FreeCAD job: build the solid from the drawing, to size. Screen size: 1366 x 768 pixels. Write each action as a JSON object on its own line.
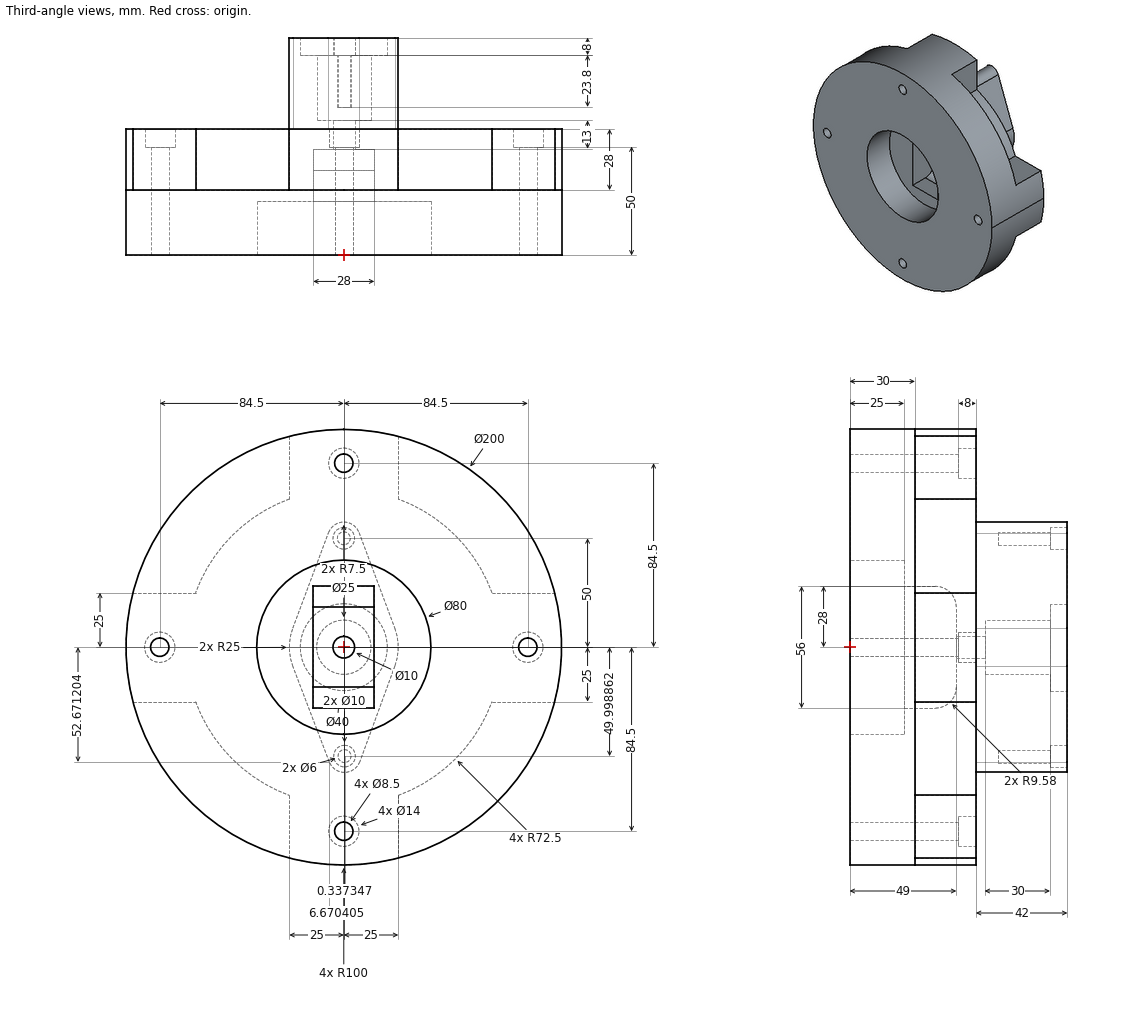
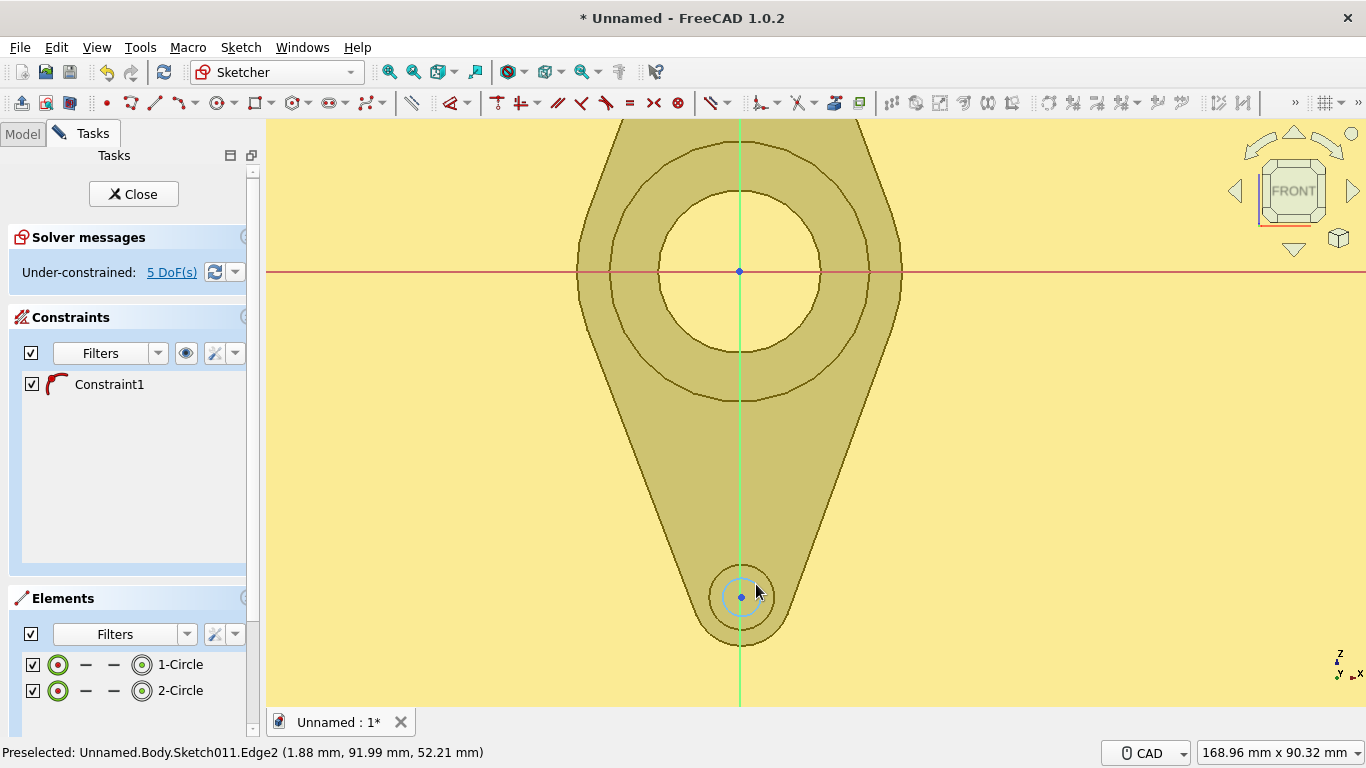
{"action": "left_click", "coordinate": [755, 584]}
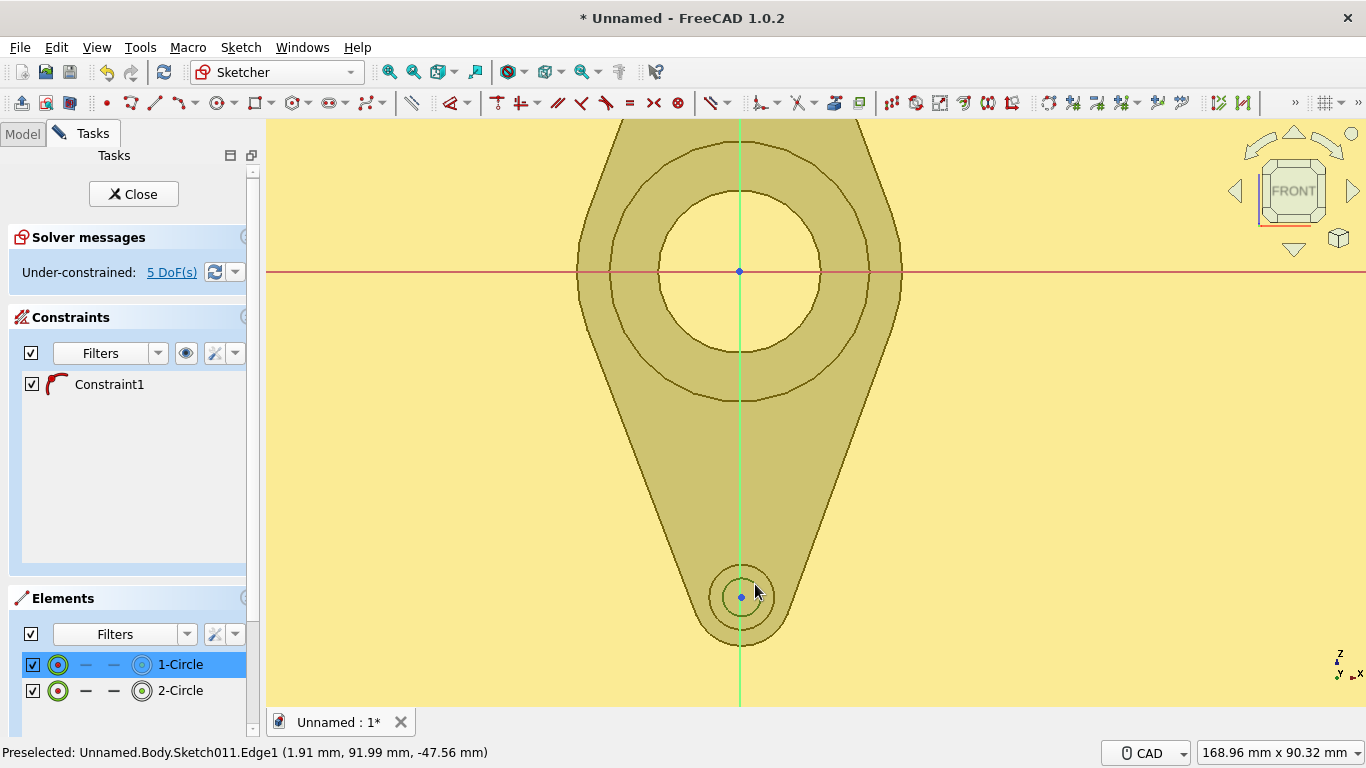
{"action": "scroll", "coordinate": [756, 585], "scroll_direction": "down", "scroll_amount": 3}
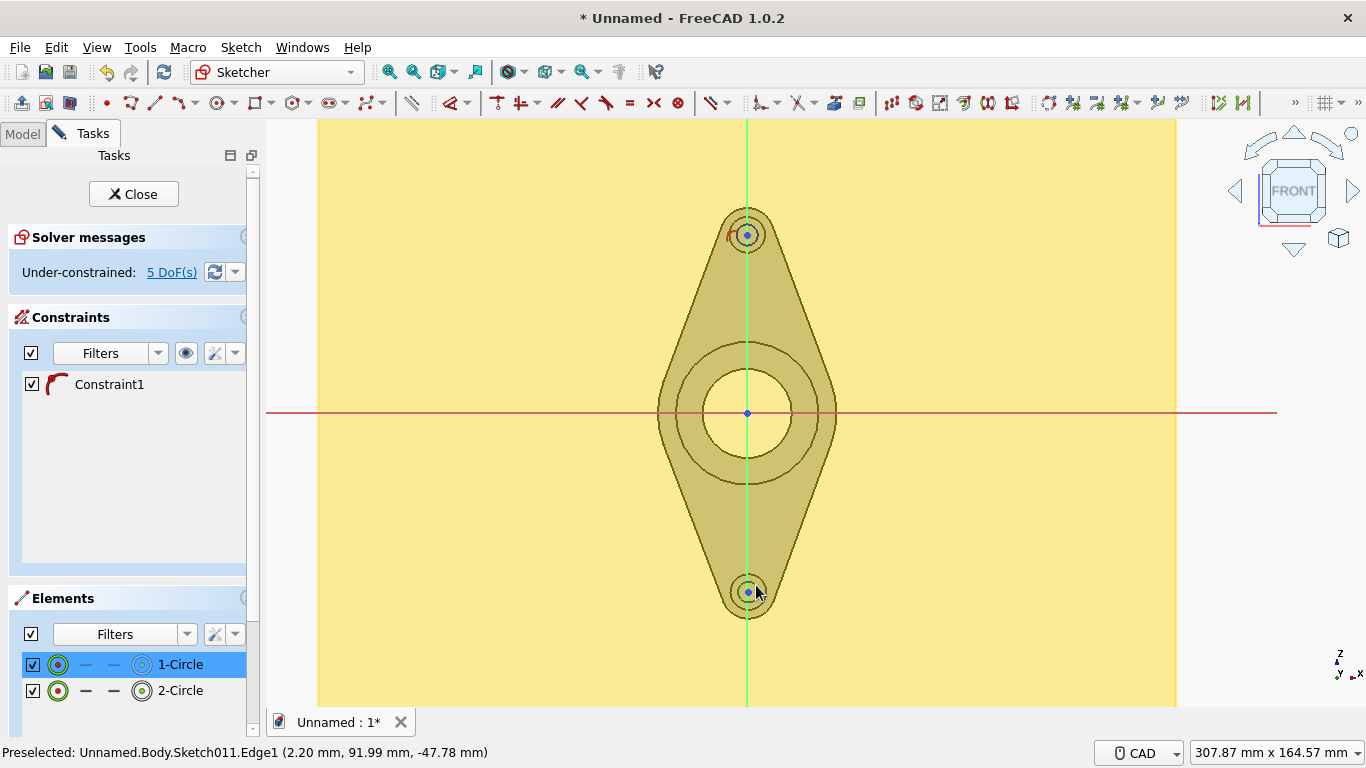
{"action": "scroll", "coordinate": [755, 228], "scroll_direction": "up", "scroll_amount": 4}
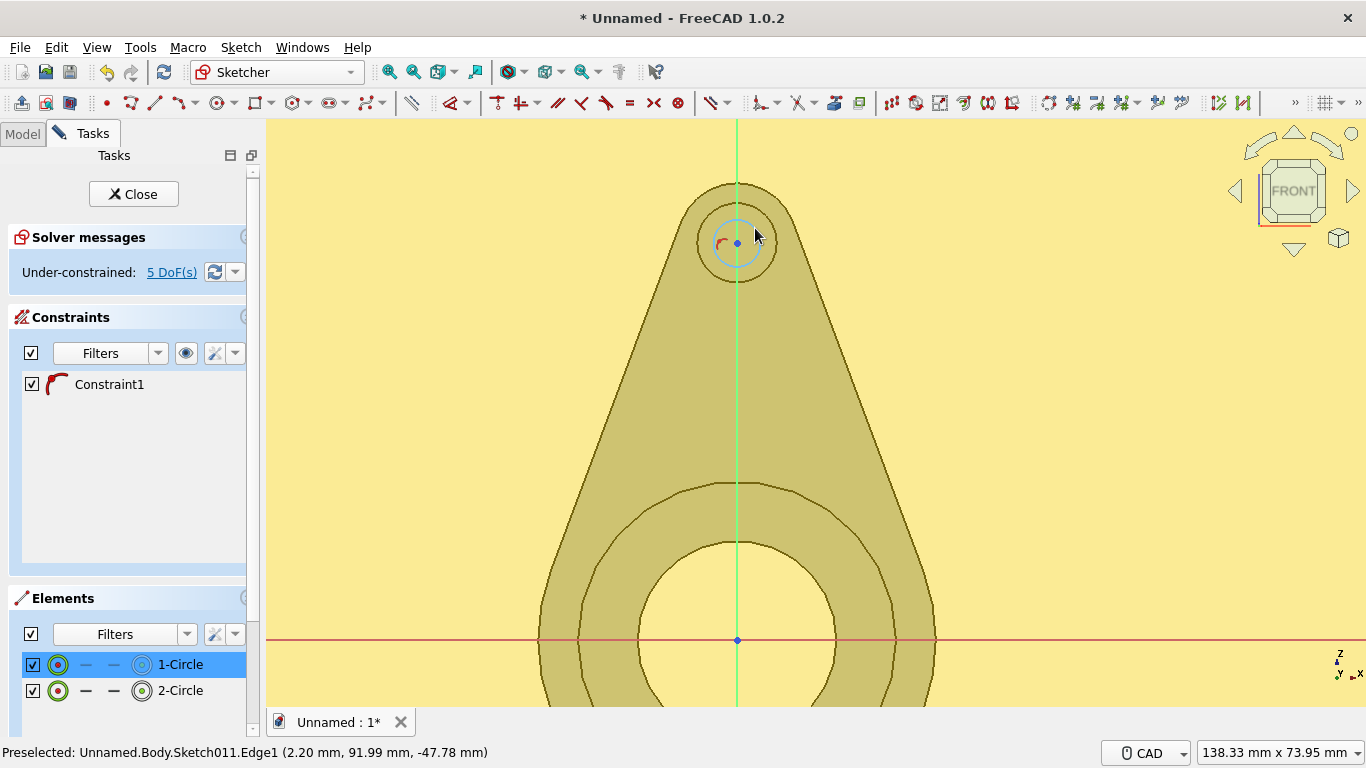
{"action": "left_click", "coordinate": [754, 227]}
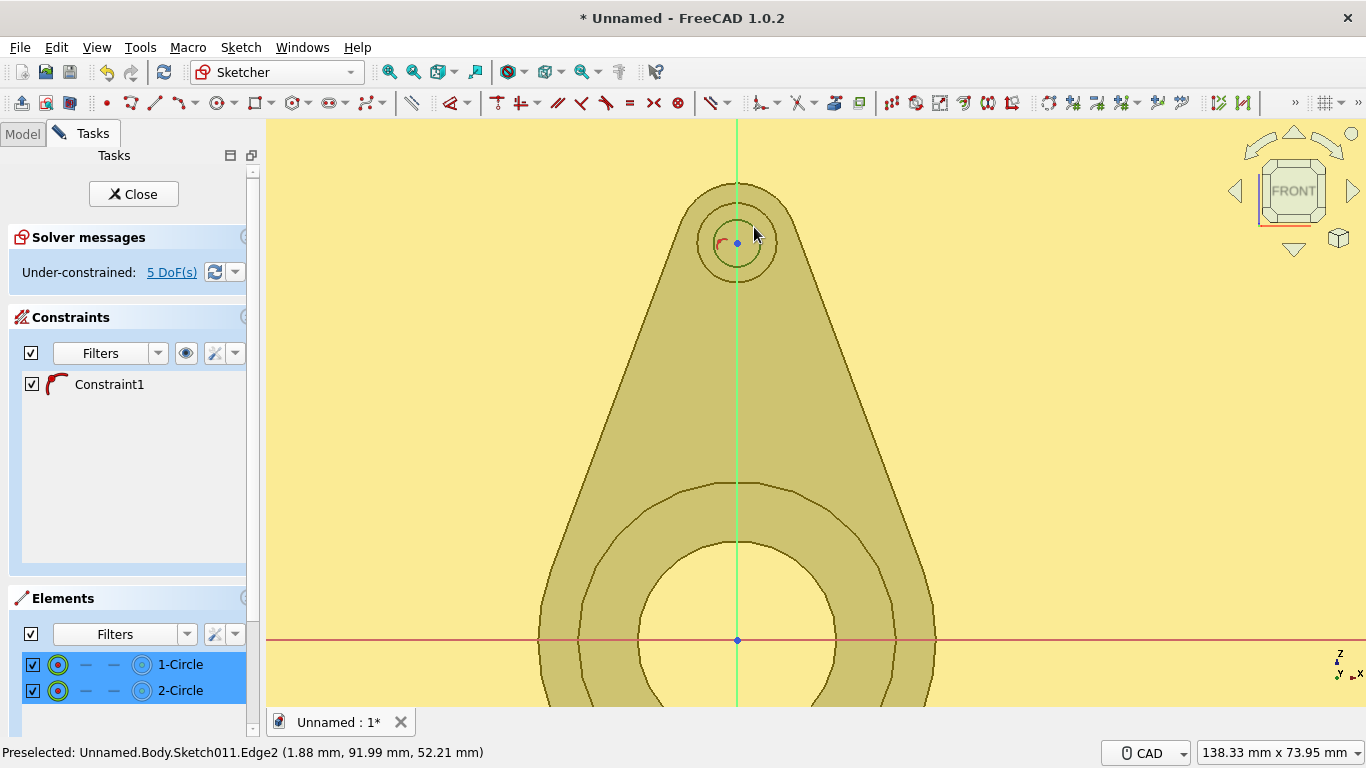
{"action": "left_click", "coordinate": [630, 104]}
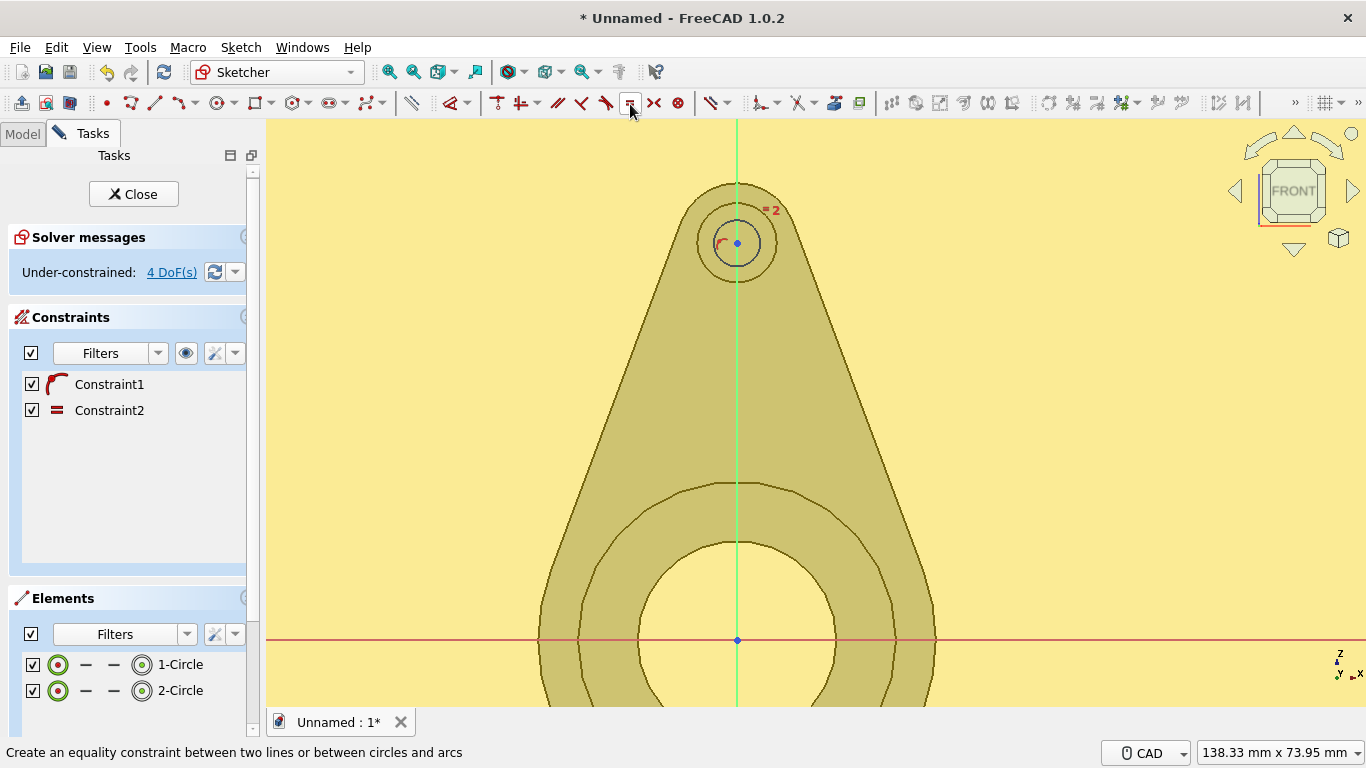
{"action": "key", "text": "d"}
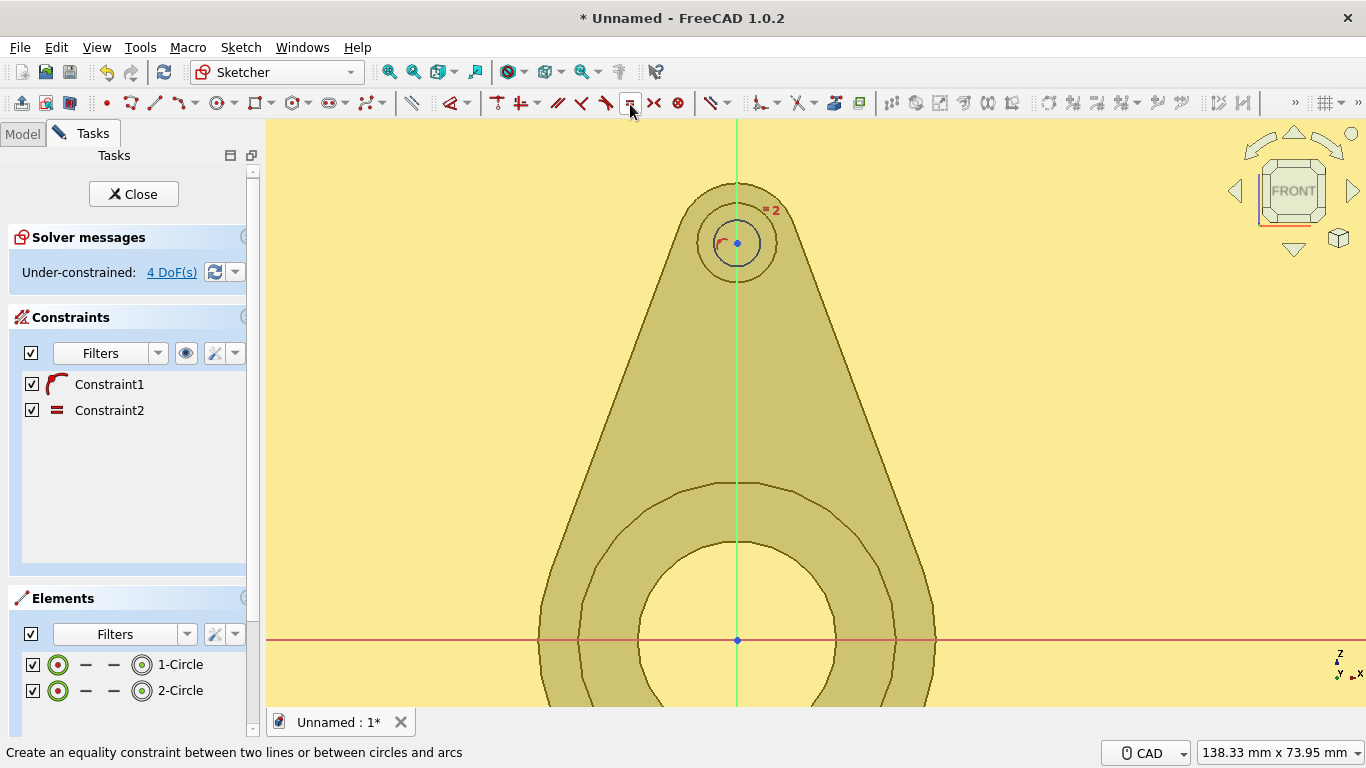
{"action": "scroll", "coordinate": [755, 227], "scroll_direction": "down", "scroll_amount": 4}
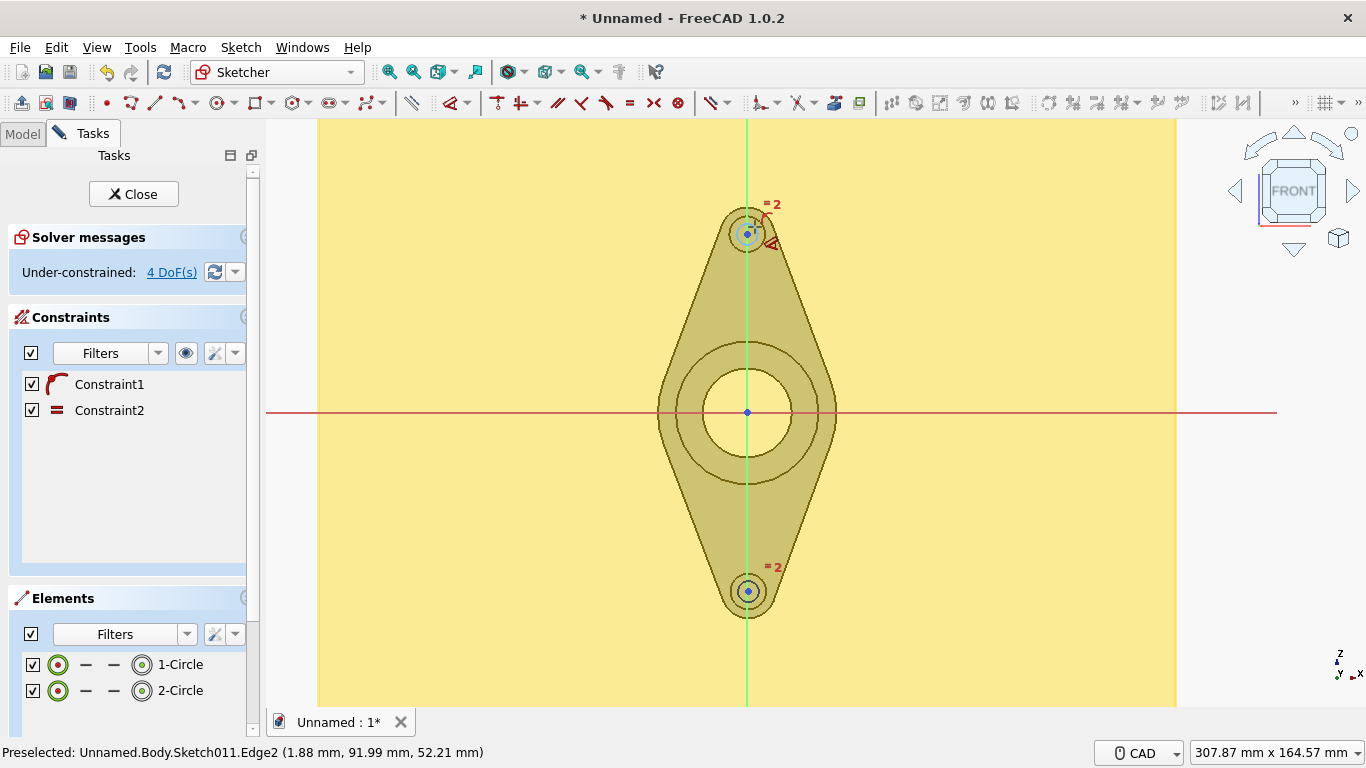
{"action": "scroll", "coordinate": [756, 584], "scroll_direction": "up", "scroll_amount": 4}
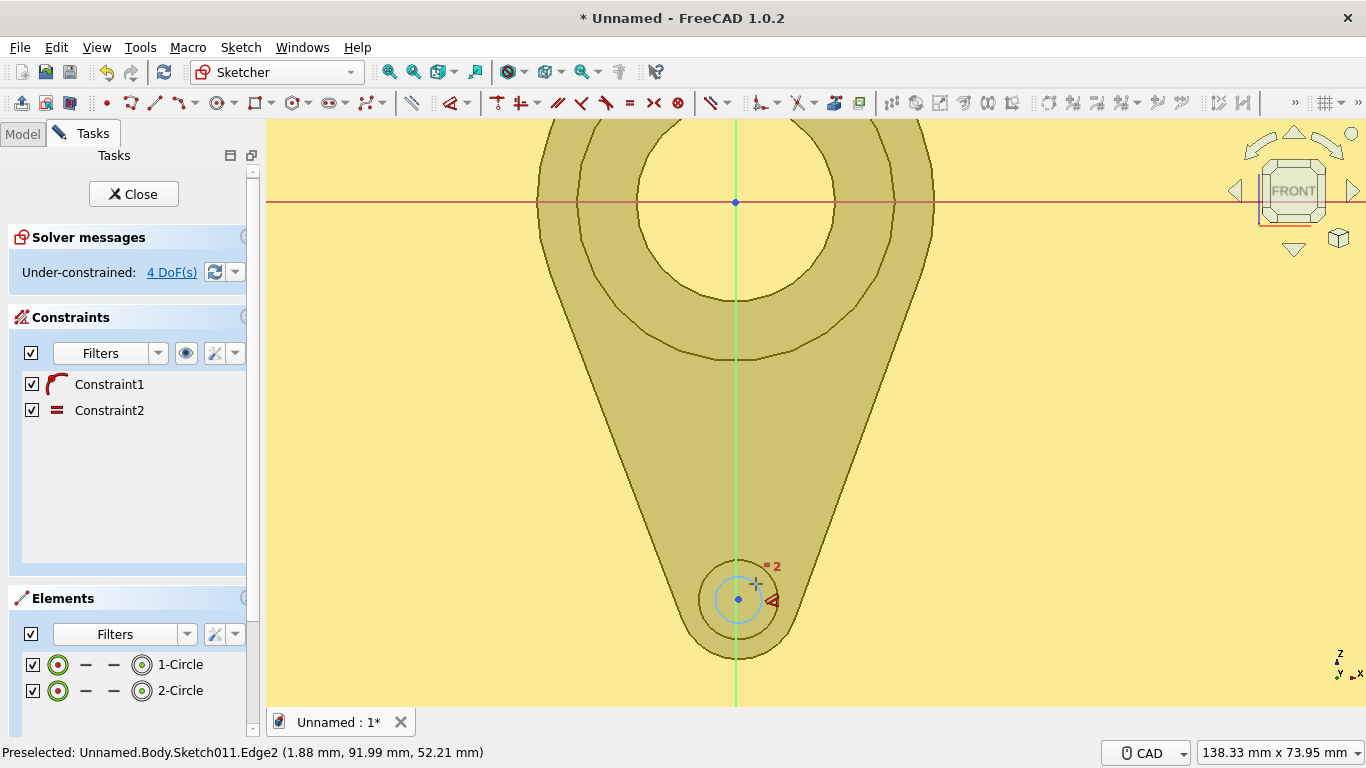
{"action": "left_click", "coordinate": [755, 583]}
{"action": "left_click", "coordinate": [777, 560]}